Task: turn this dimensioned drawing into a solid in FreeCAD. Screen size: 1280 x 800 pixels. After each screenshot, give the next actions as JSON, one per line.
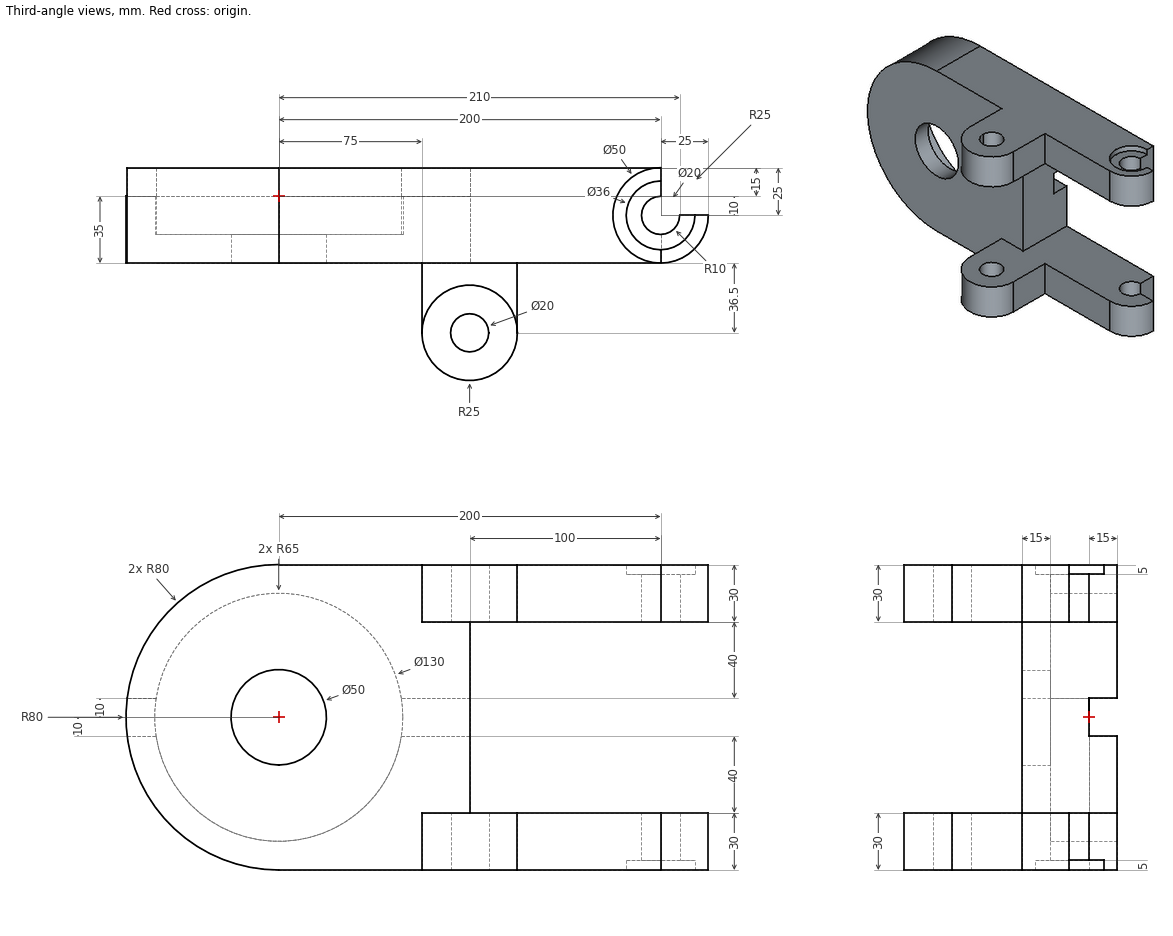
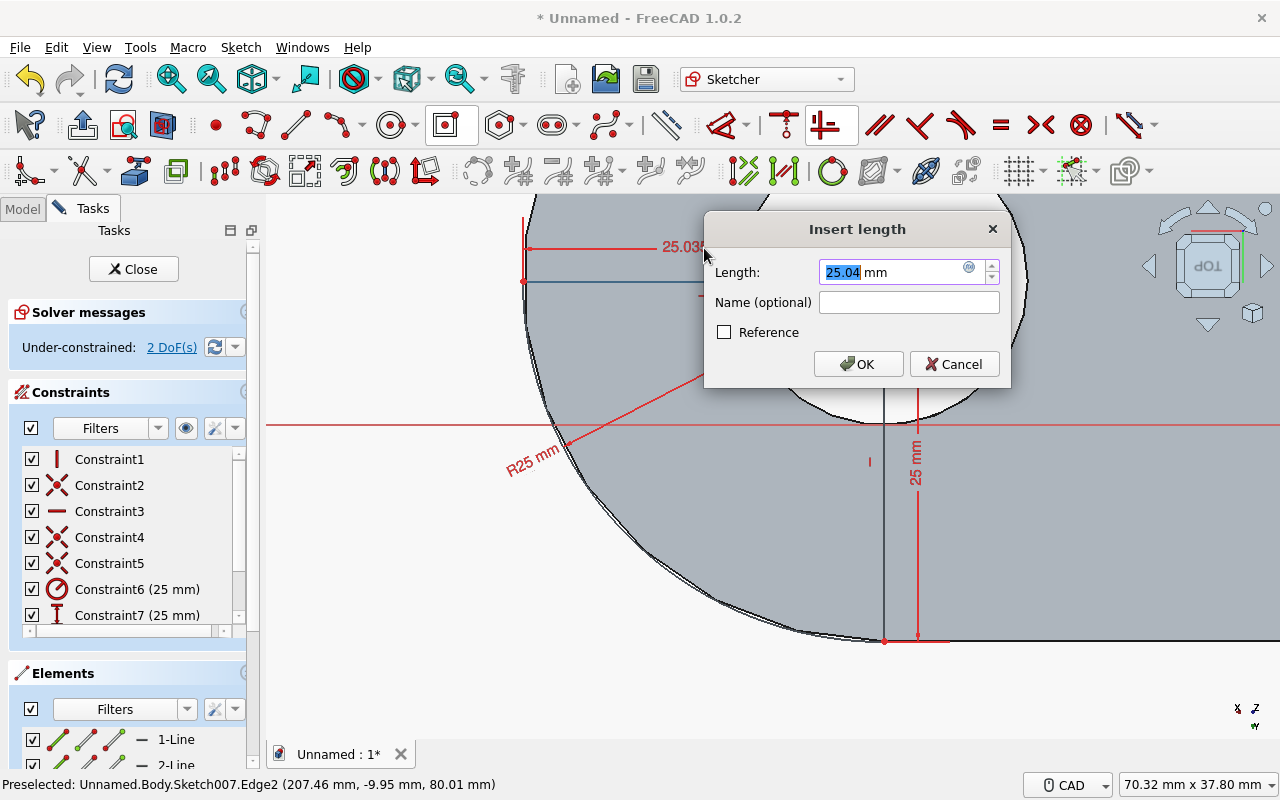
{"action": "type", "text": "25"}
{"action": "key", "text": "Return"}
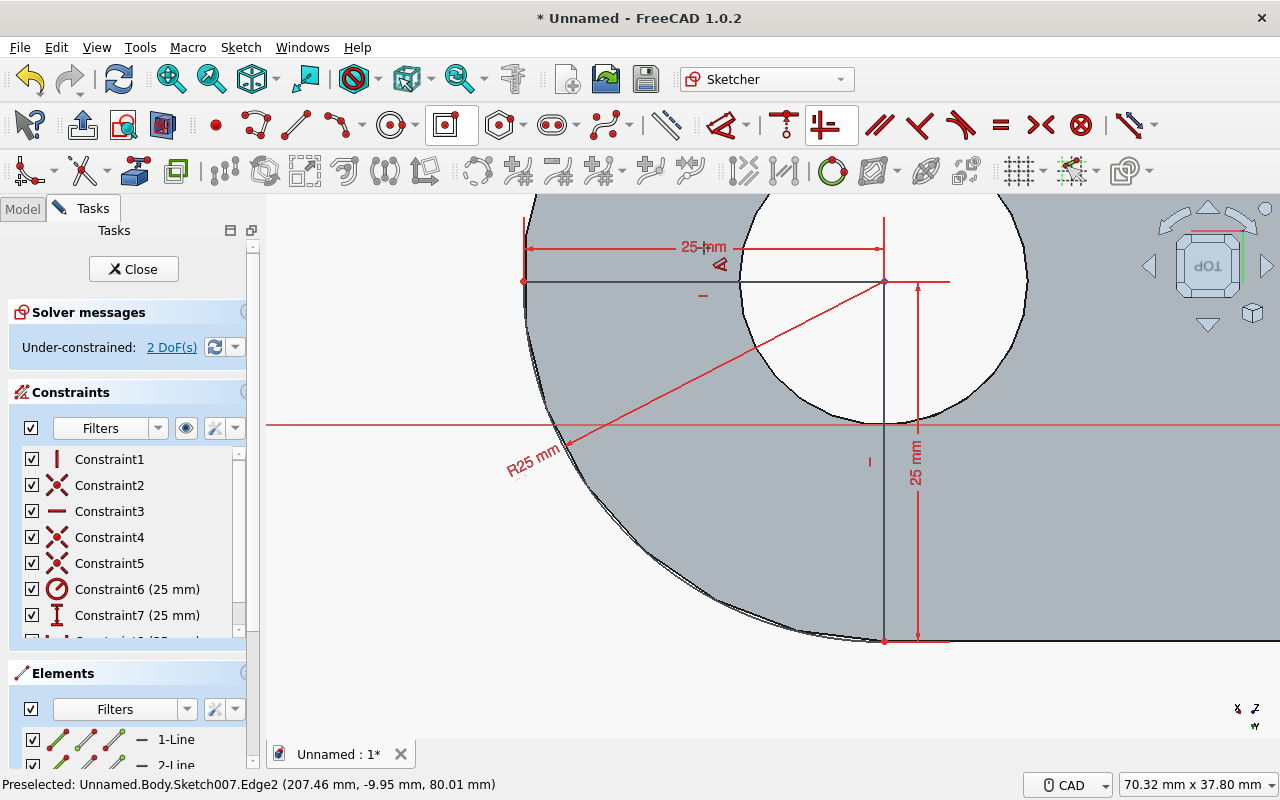
{"action": "left_click", "coordinate": [884, 642]}
{"action": "left_click", "coordinate": [850, 533]}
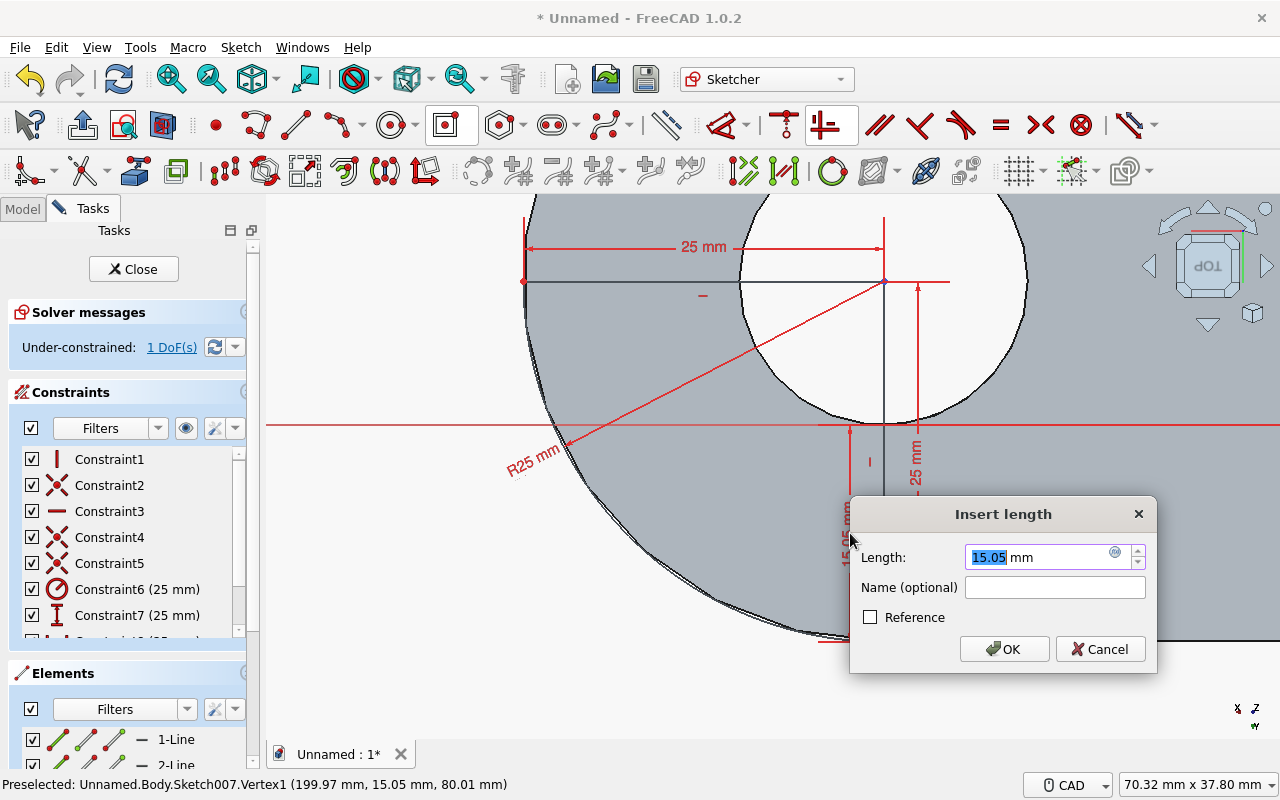
{"action": "type", "text": "15"}
{"action": "key", "text": "Return"}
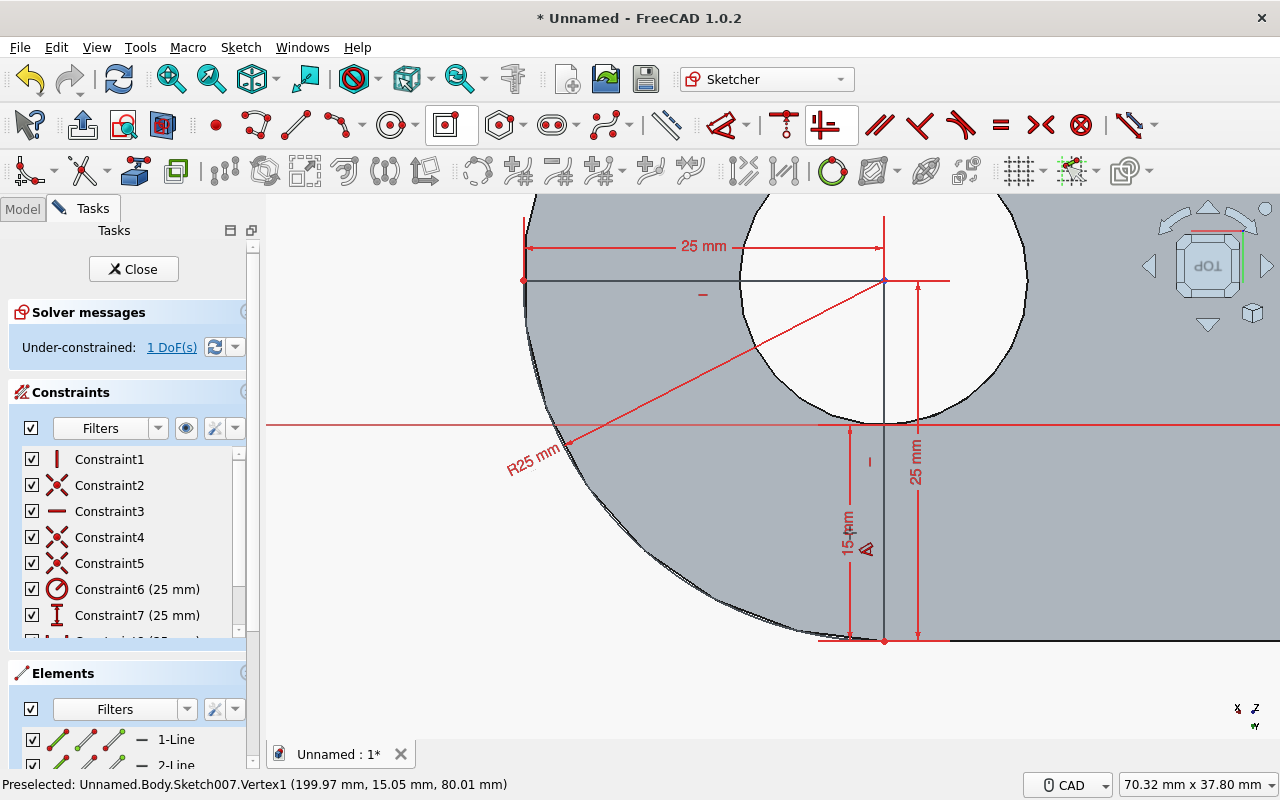
{"action": "left_click", "coordinate": [884, 641]}
{"action": "left_click", "coordinate": [999, 675]}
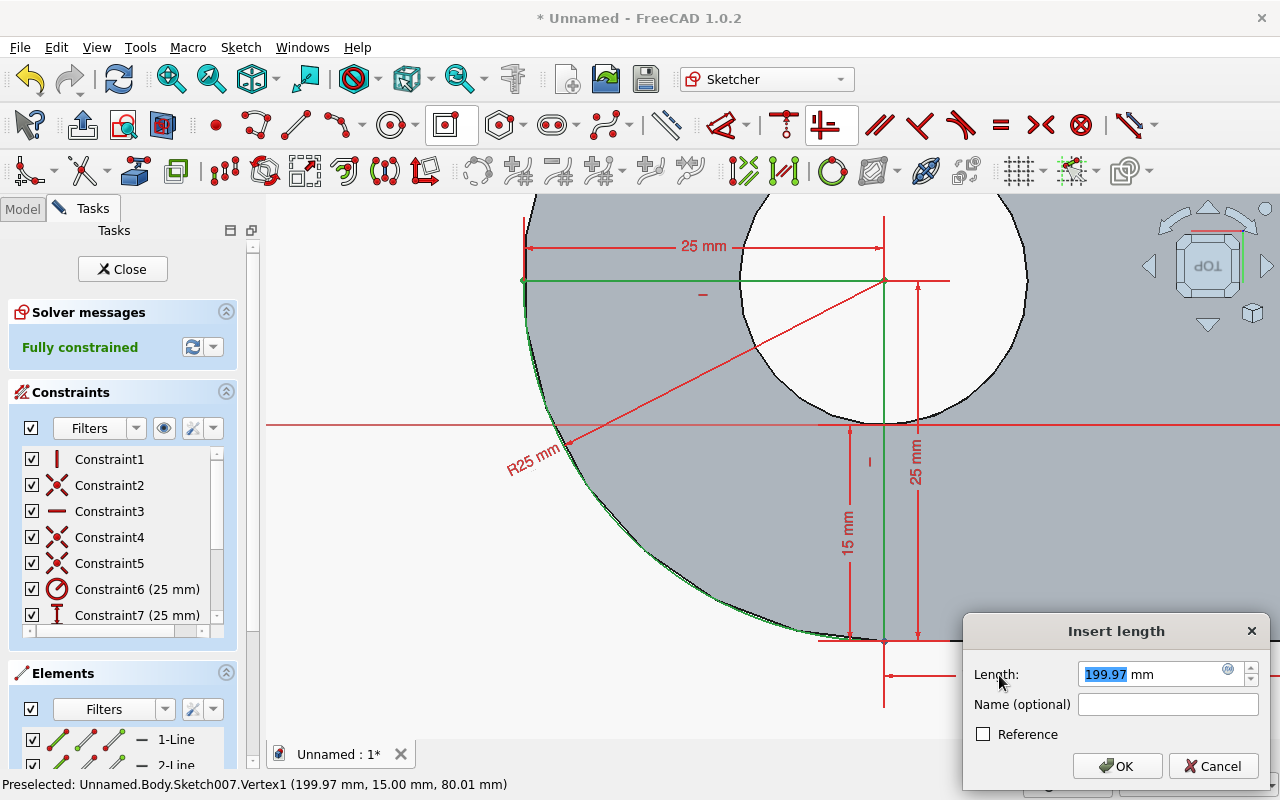
{"action": "type", "text": "200"}
{"action": "key", "text": "Return"}
{"action": "key", "text": "Escape"}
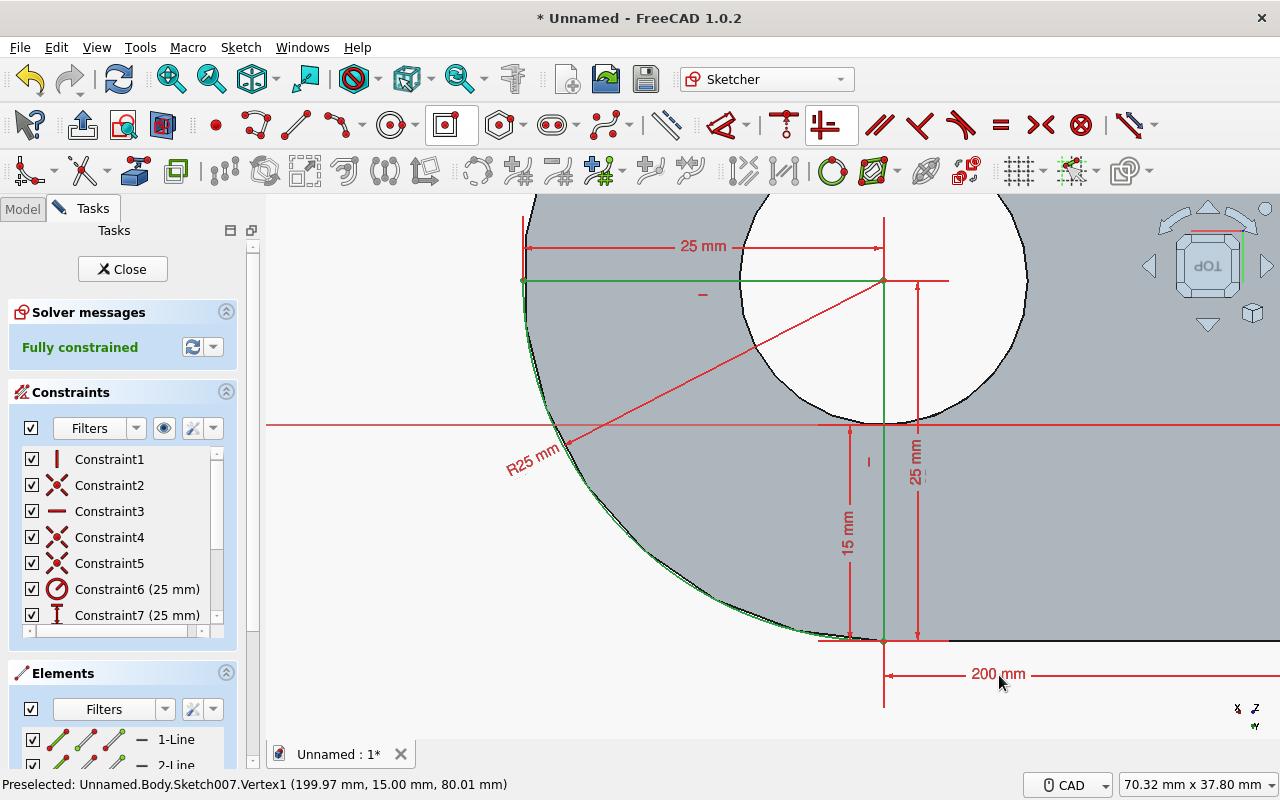
{"action": "left_click", "coordinate": [123, 269]}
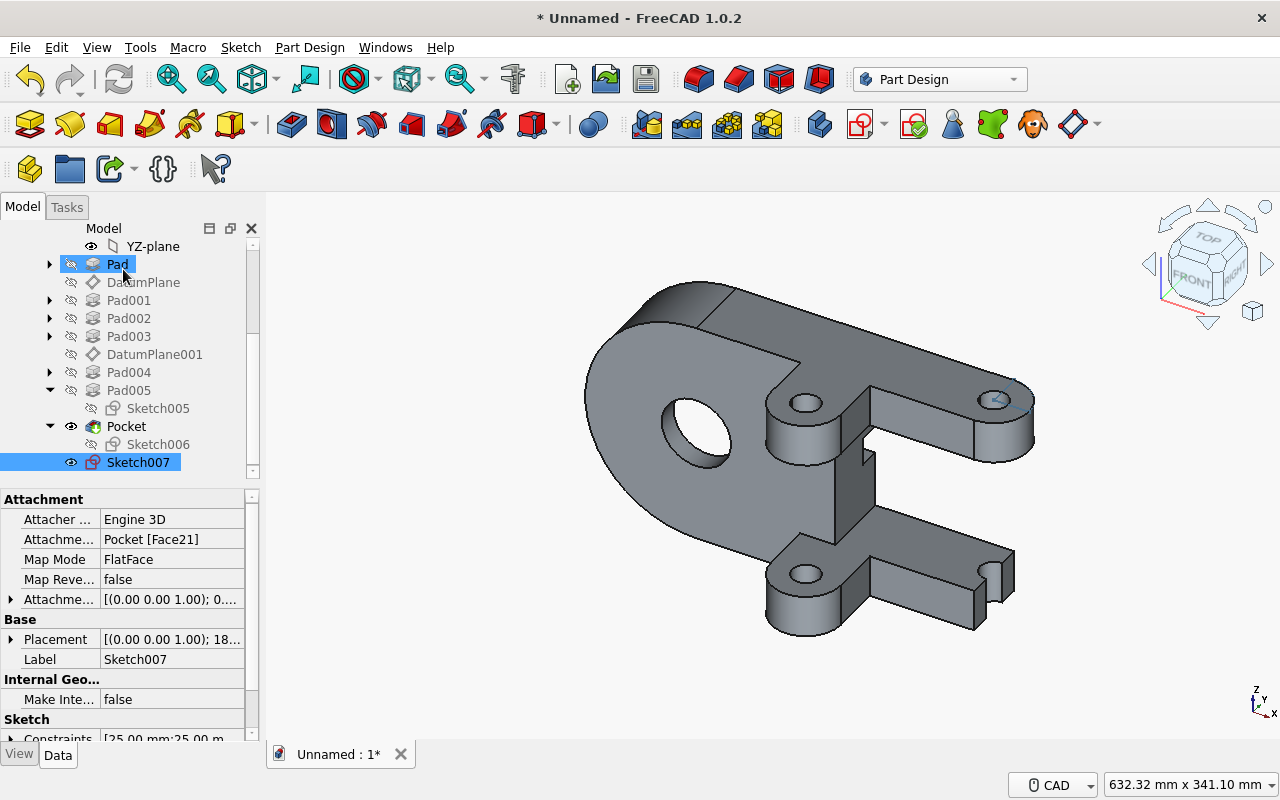
{"action": "left_click", "coordinate": [292, 124]}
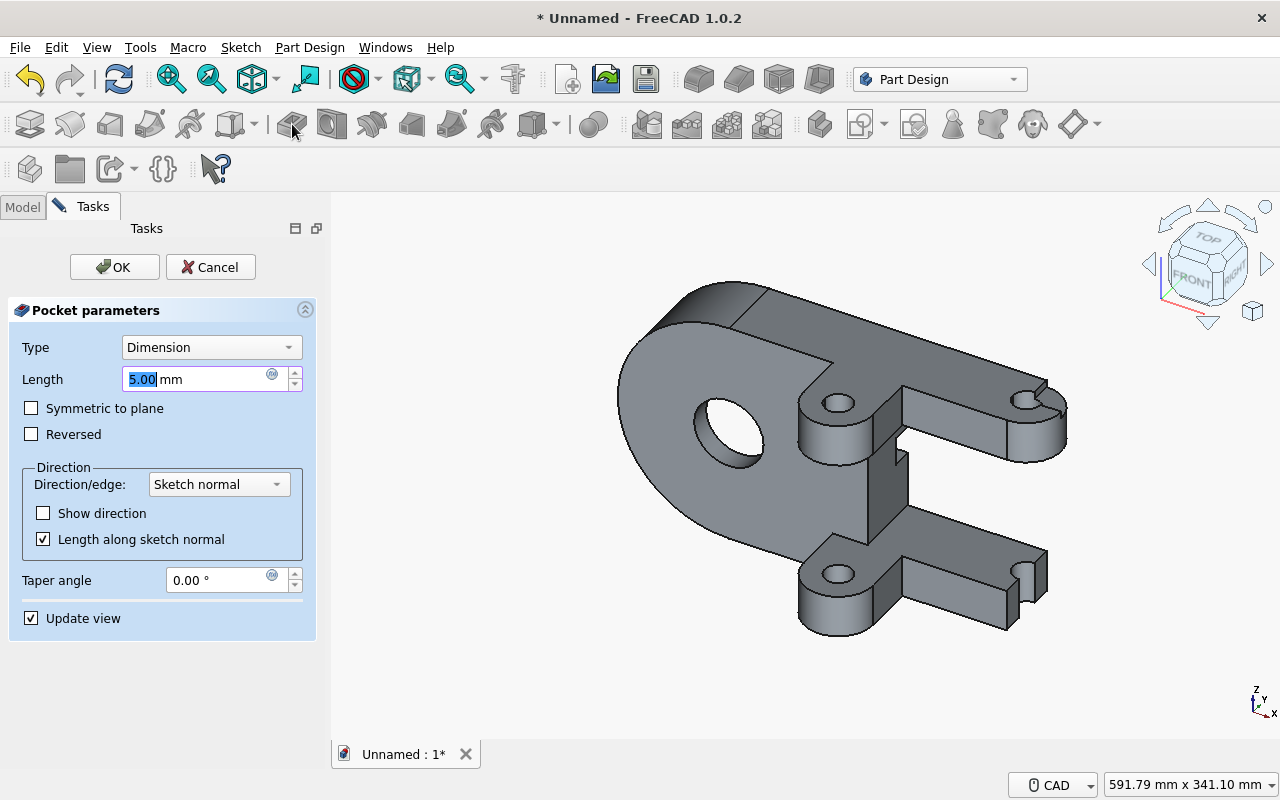
{"action": "type", "text": "200"}
{"action": "key", "text": "Tab"}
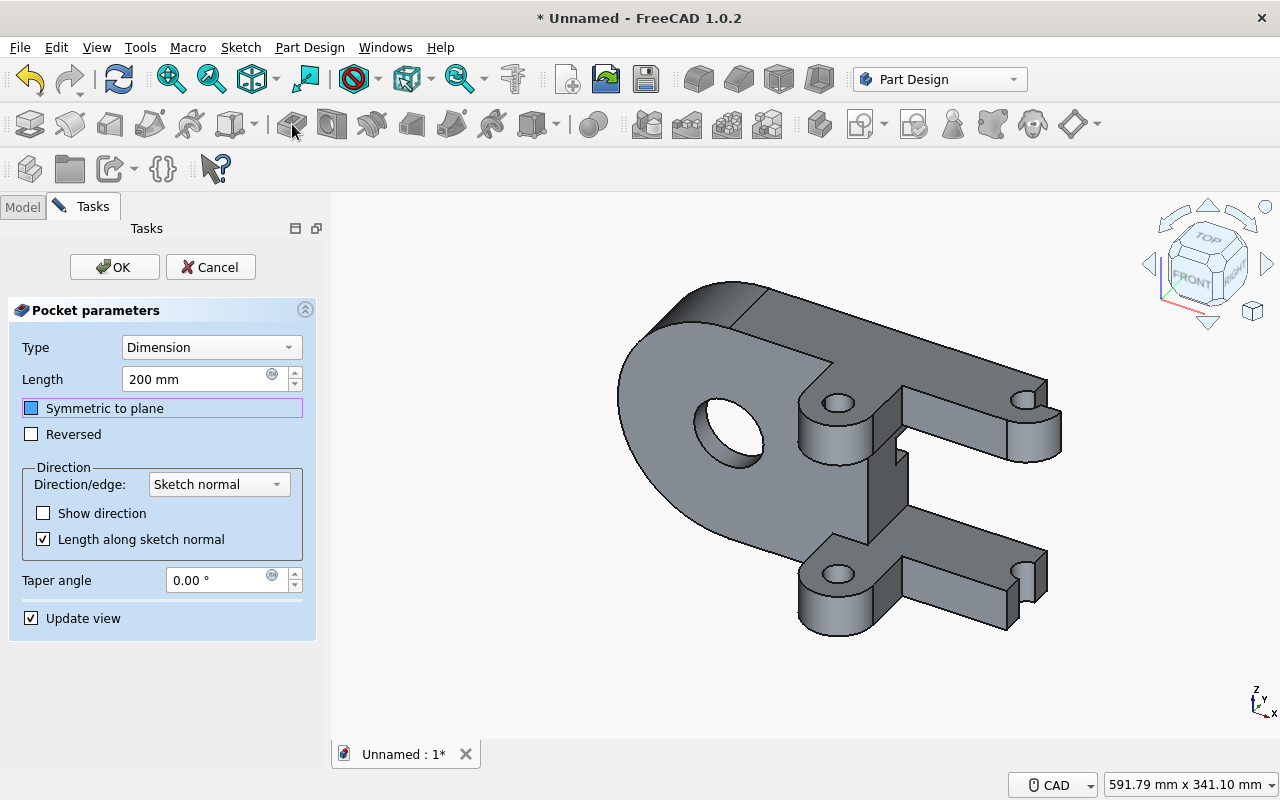
{"action": "left_click", "coordinate": [115, 267]}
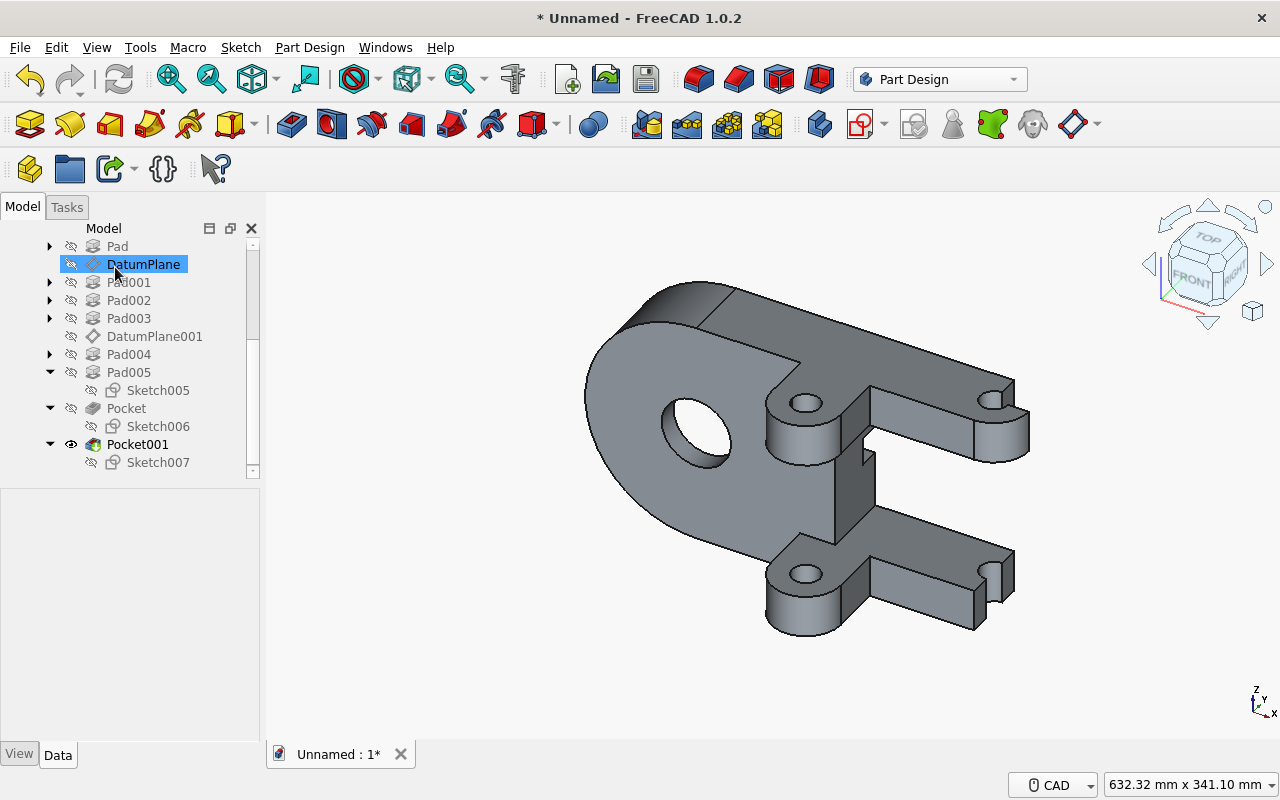
{"action": "left_click", "coordinate": [918, 373]}